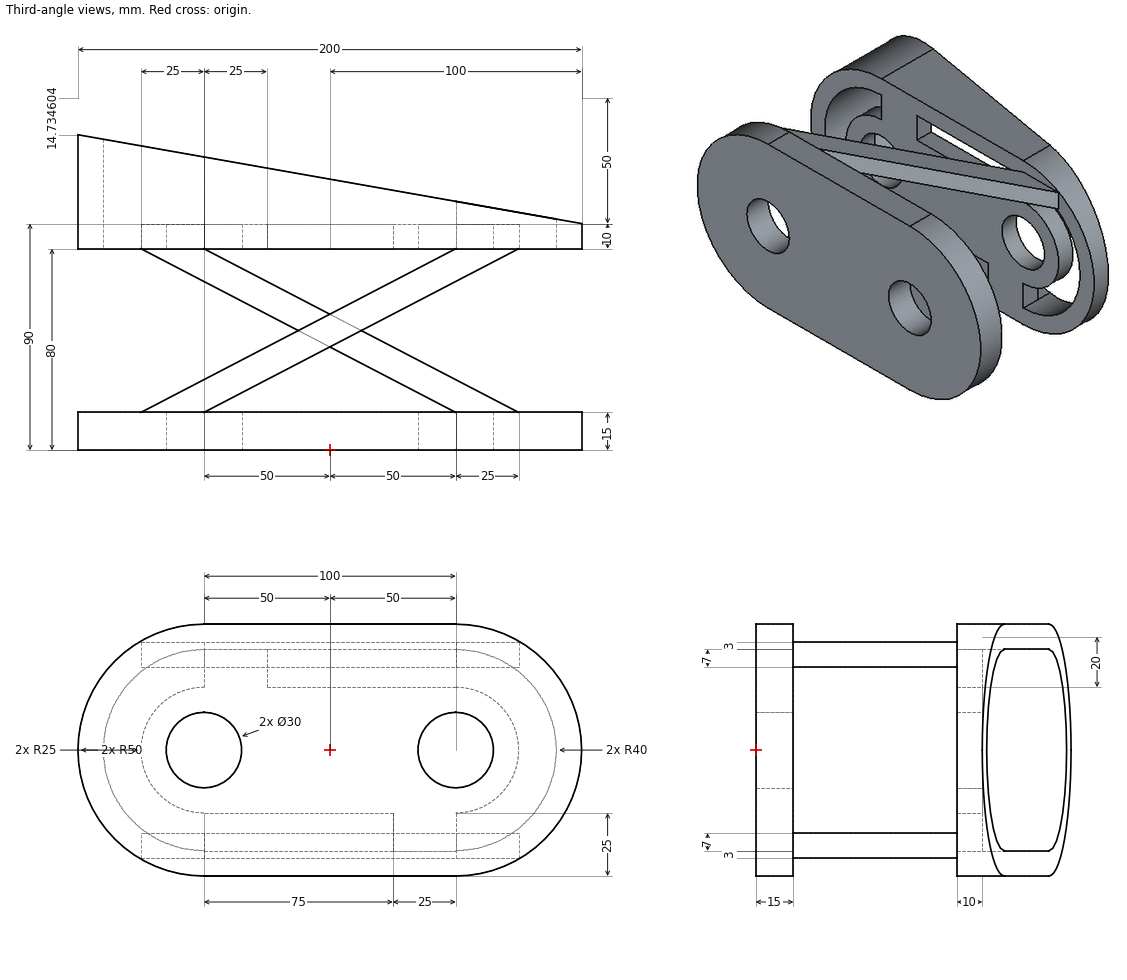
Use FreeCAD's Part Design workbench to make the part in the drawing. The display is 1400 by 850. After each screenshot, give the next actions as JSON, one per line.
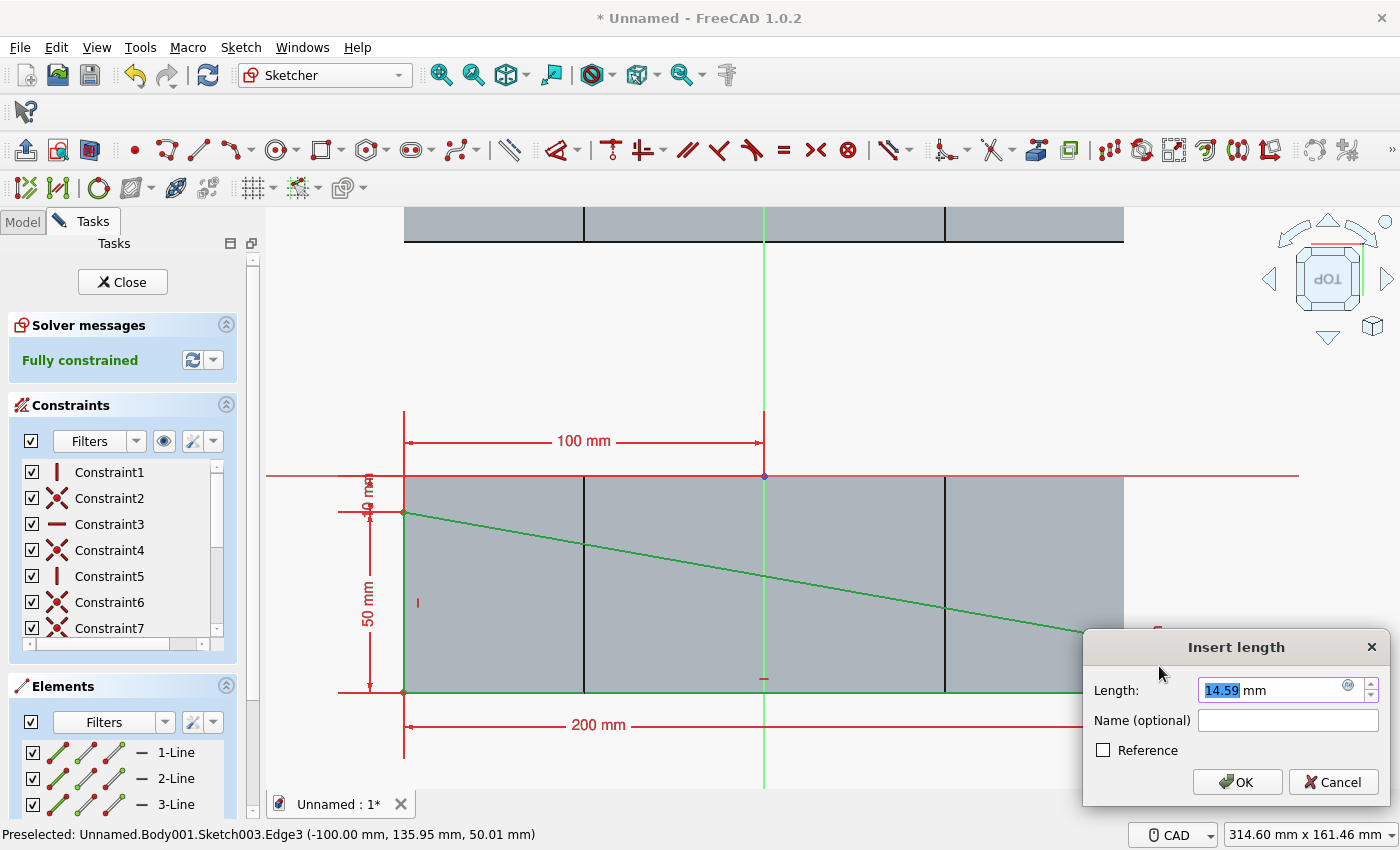
{"action": "type", "text": "14.734604"}
{"action": "key", "text": "Return"}
{"action": "key", "text": "Escape"}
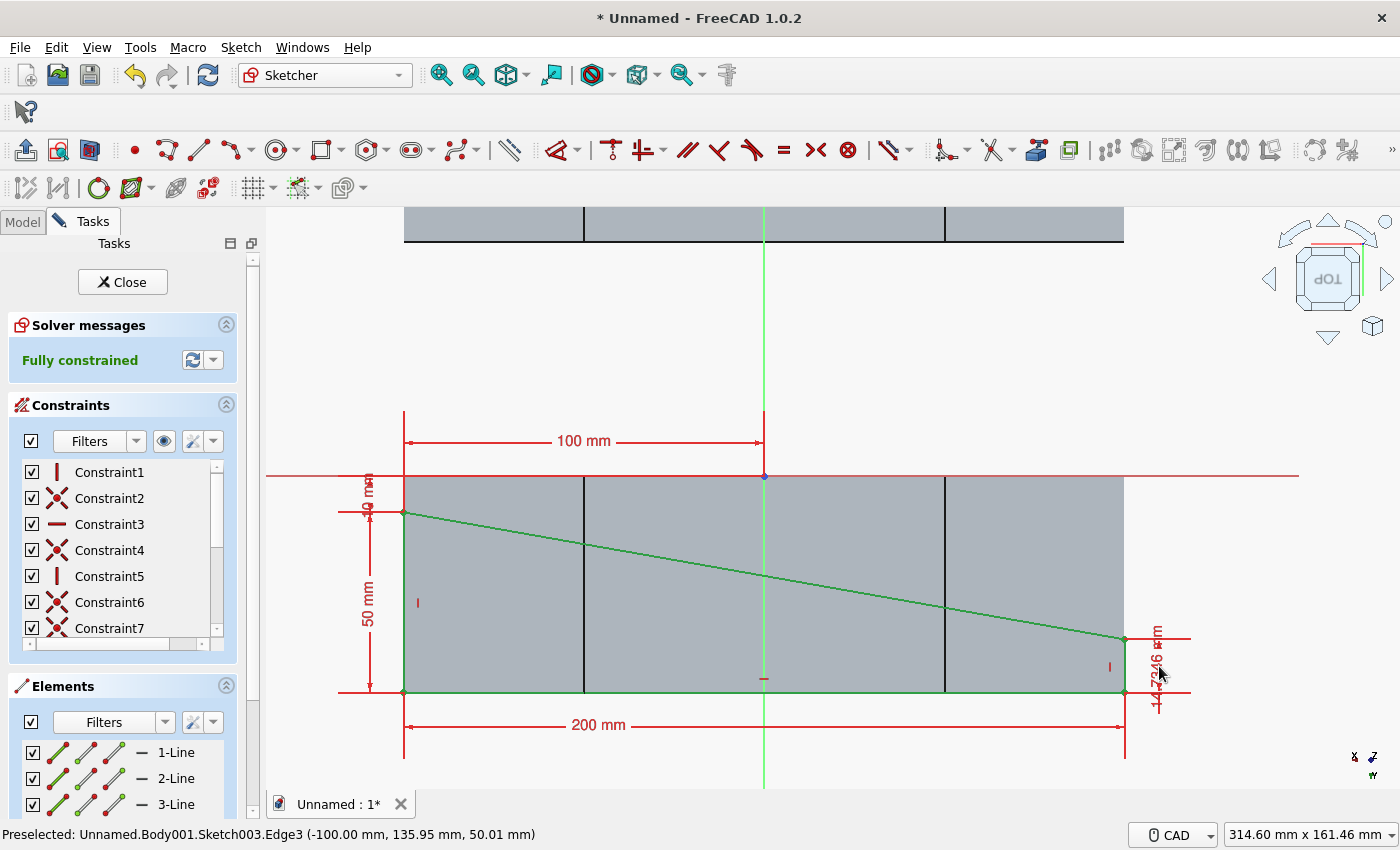
{"action": "left_click", "coordinate": [123, 282]}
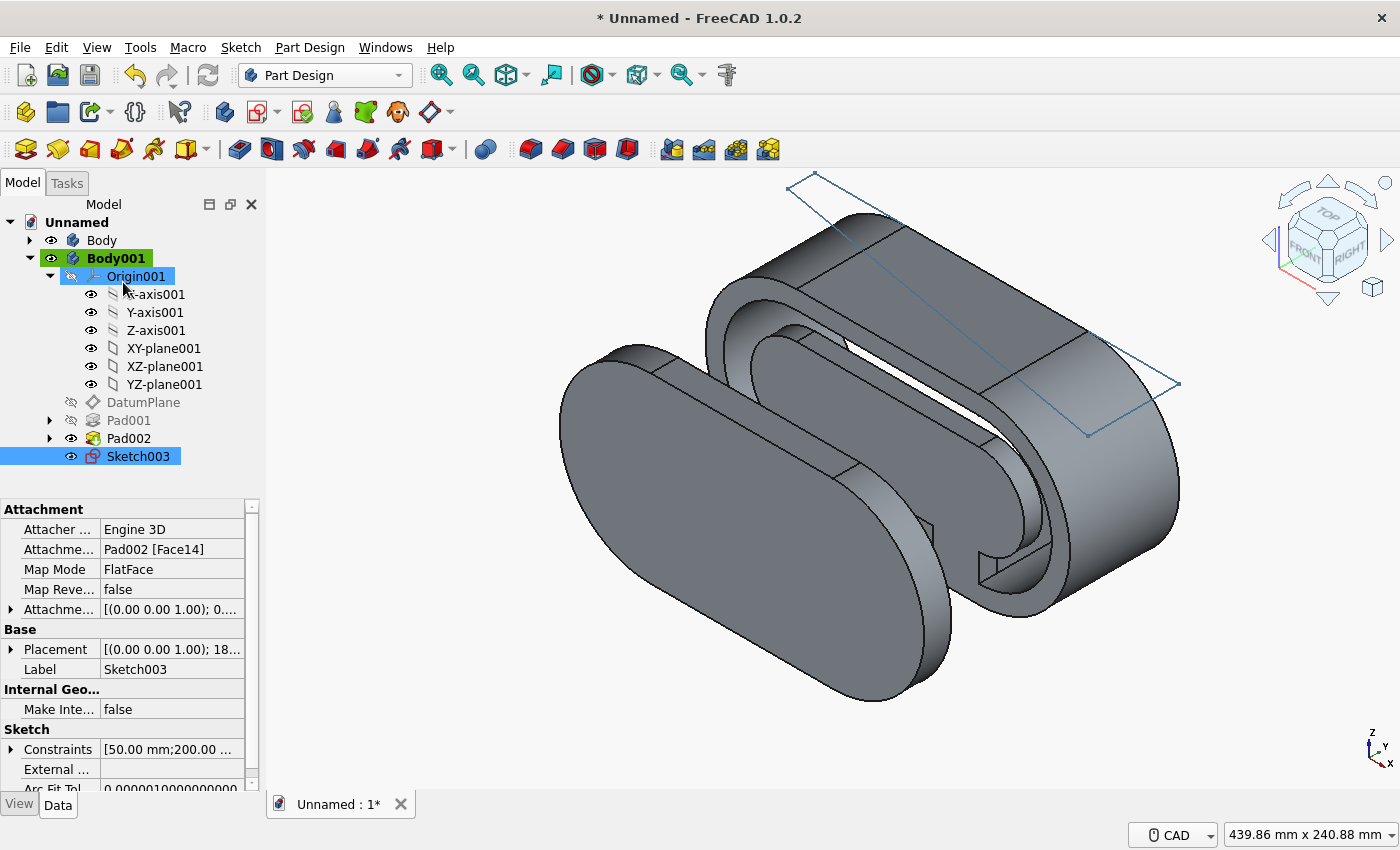
{"action": "left_click", "coordinate": [240, 150]}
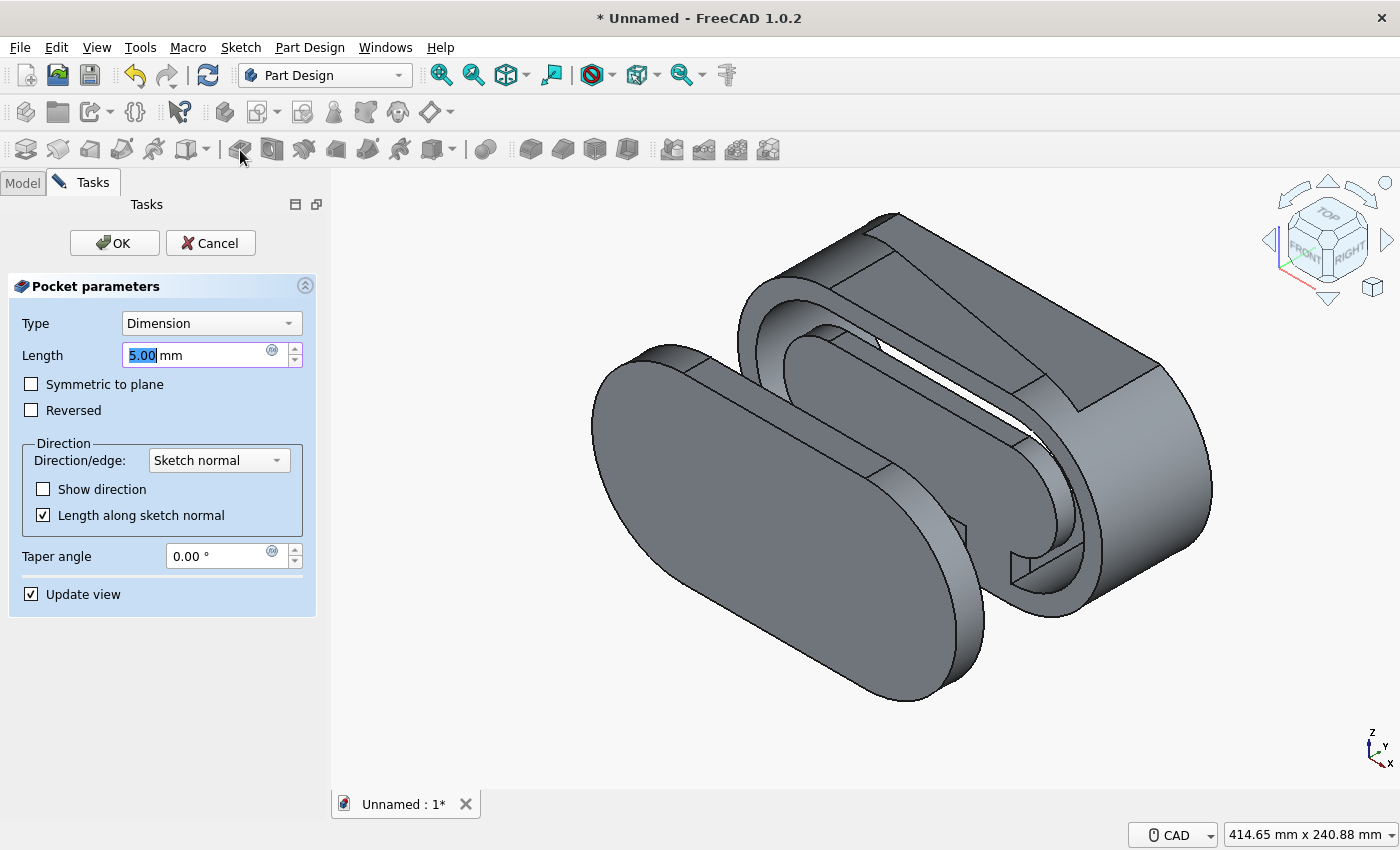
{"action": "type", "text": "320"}
{"action": "key", "text": "Tab"}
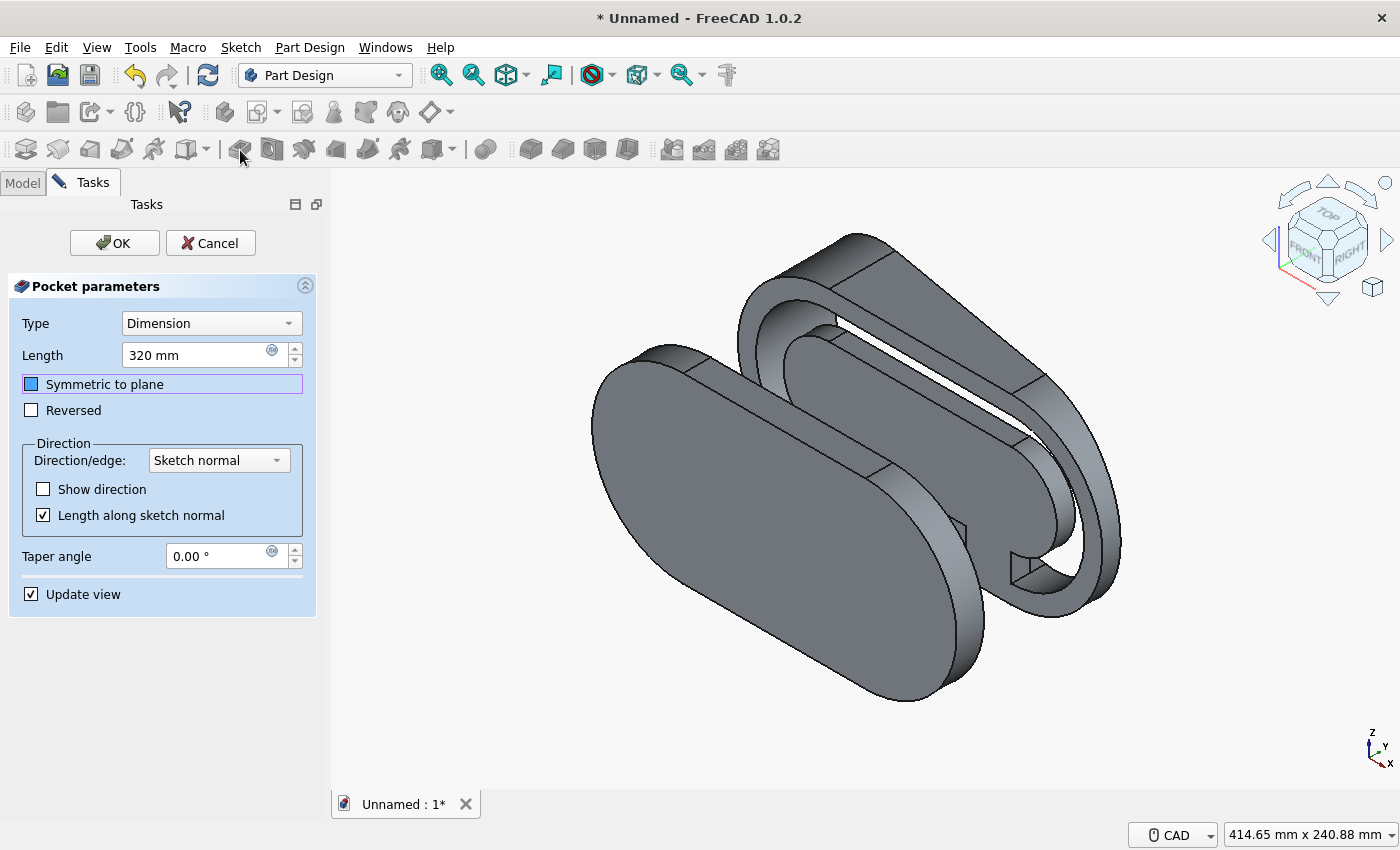
{"action": "left_click", "coordinate": [30, 384]}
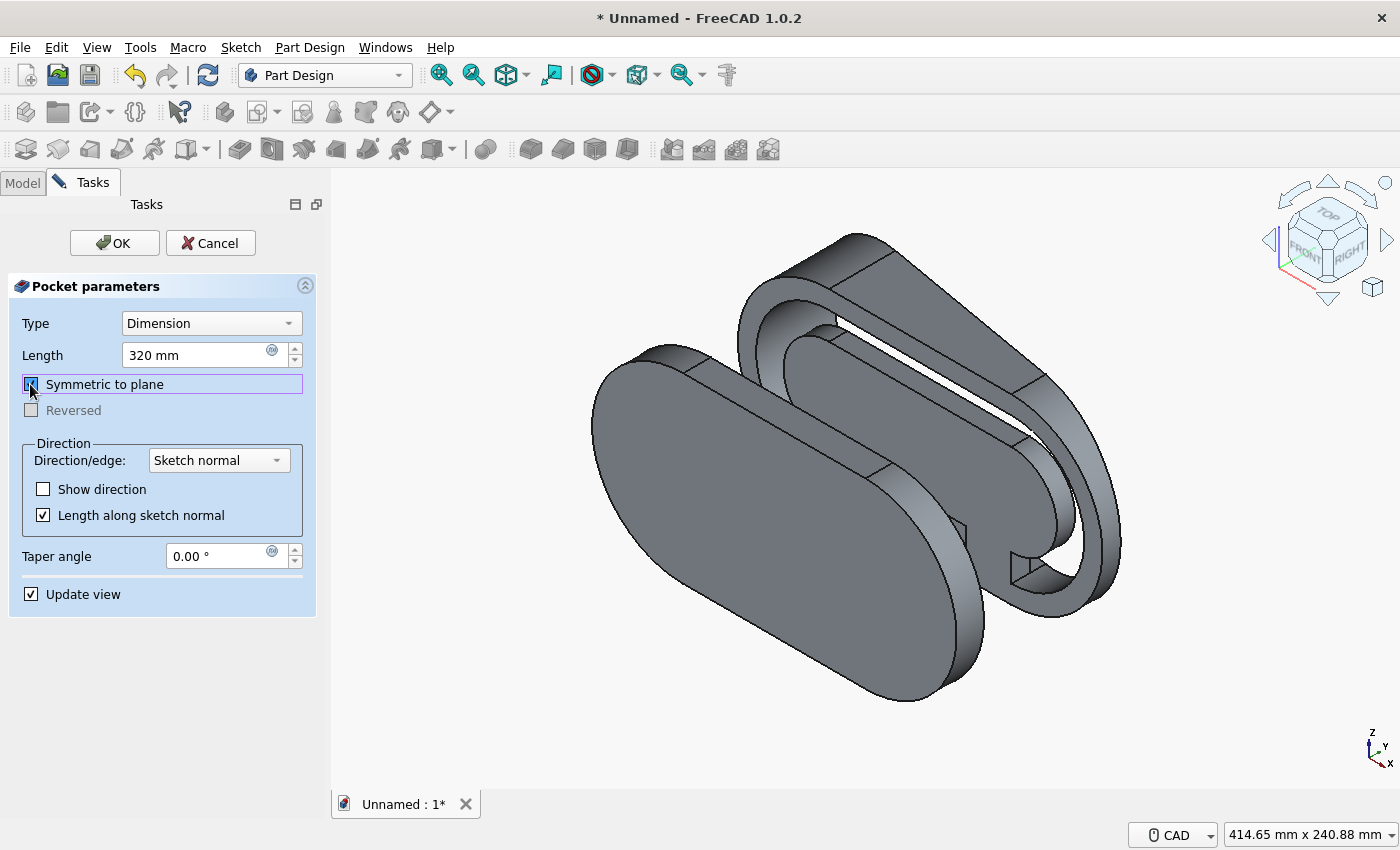
{"action": "left_click", "coordinate": [115, 243]}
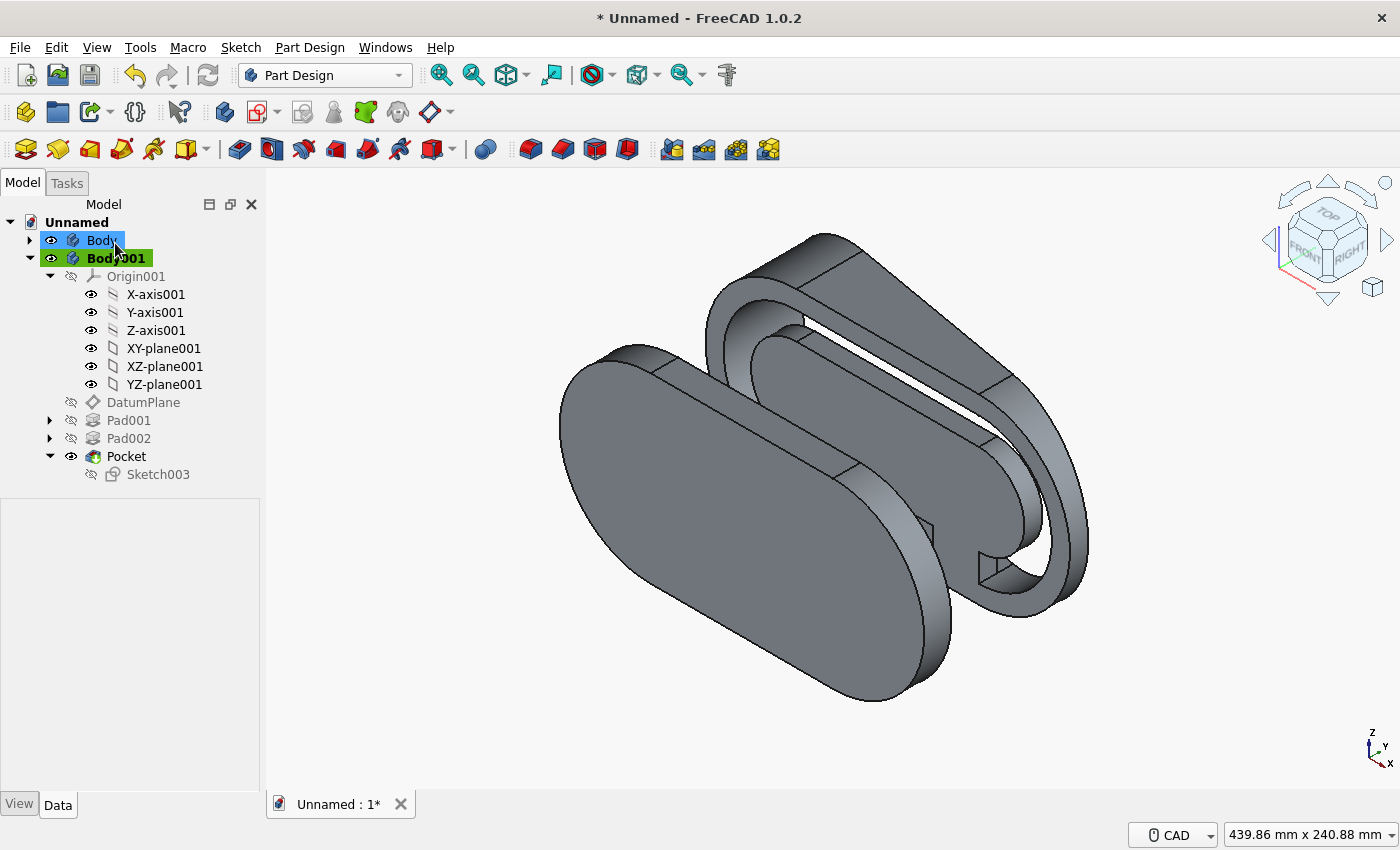
{"action": "left_click", "coordinate": [136, 348]}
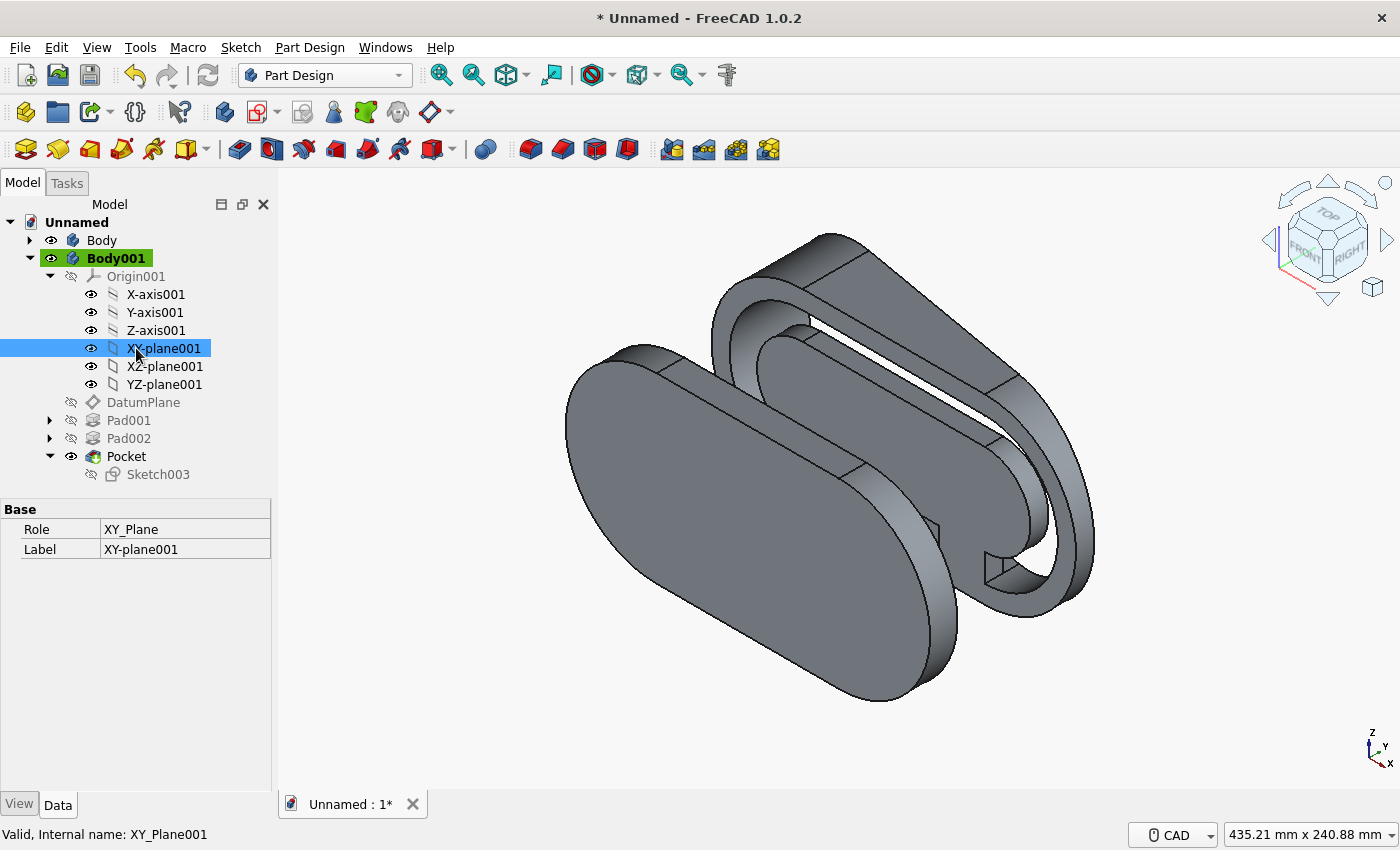
{"action": "left_click", "coordinate": [430, 112]}